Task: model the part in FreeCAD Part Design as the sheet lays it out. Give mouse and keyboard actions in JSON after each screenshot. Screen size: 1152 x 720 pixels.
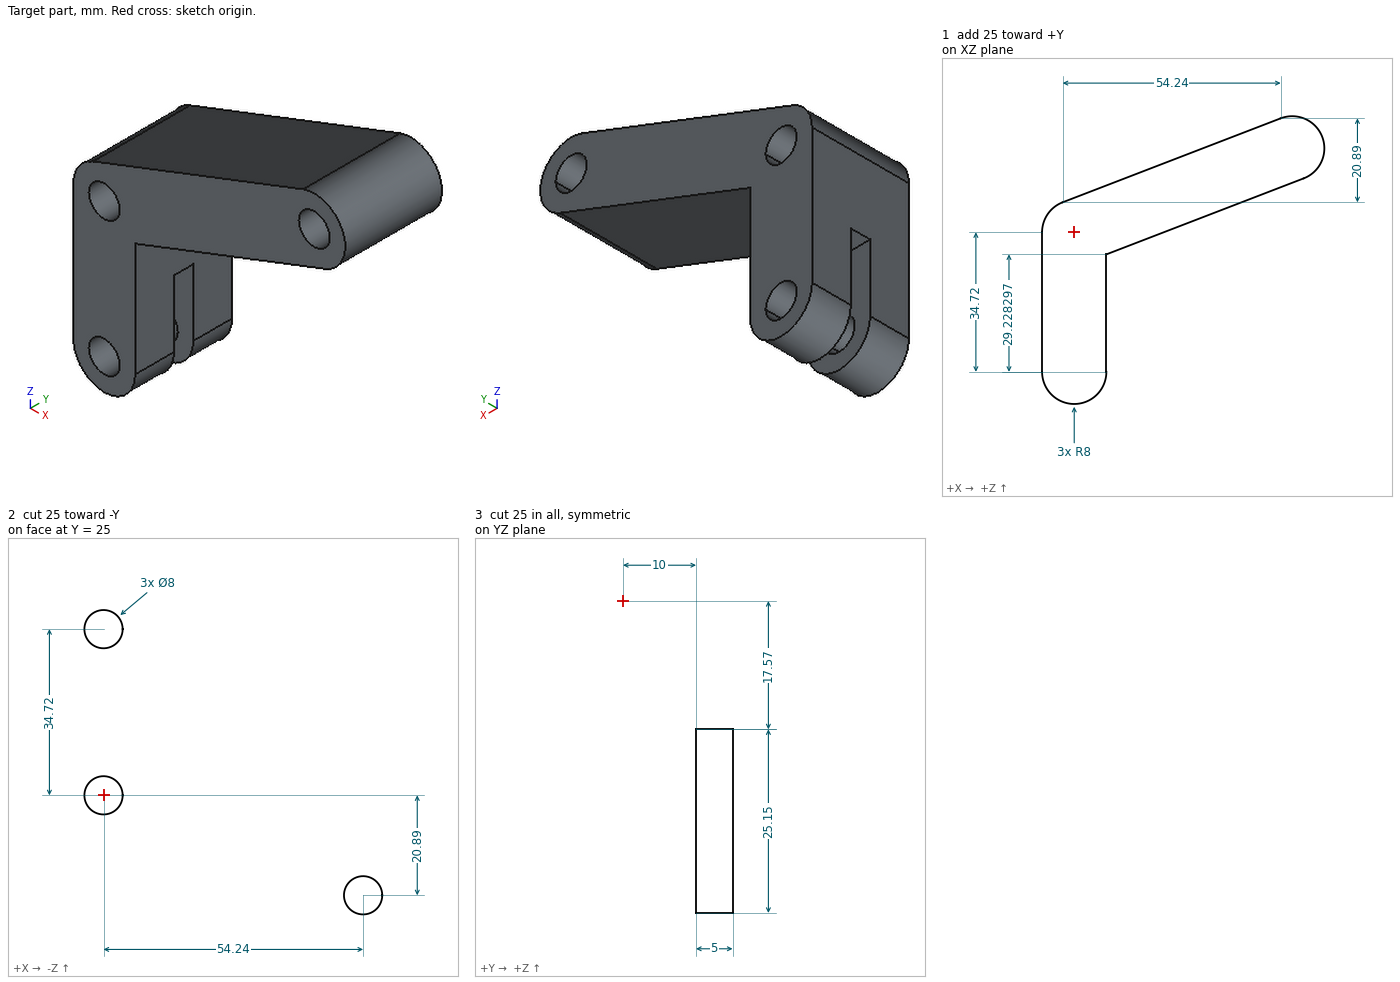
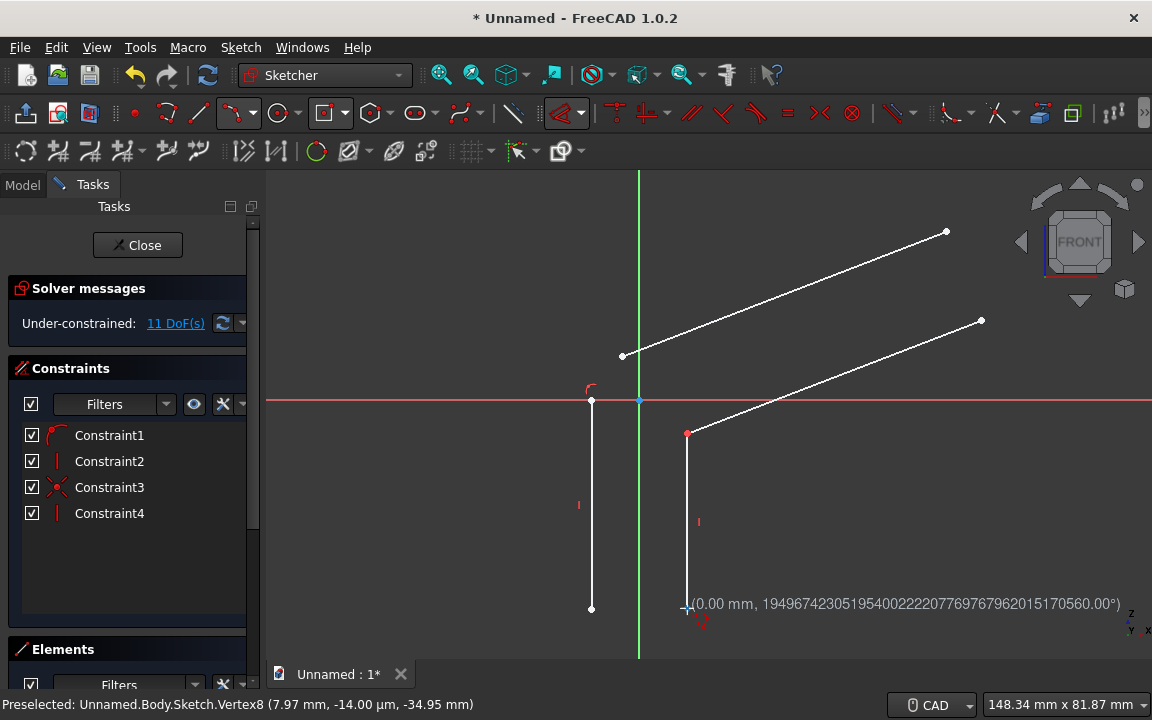
{"action": "key", "text": "g 3 a"}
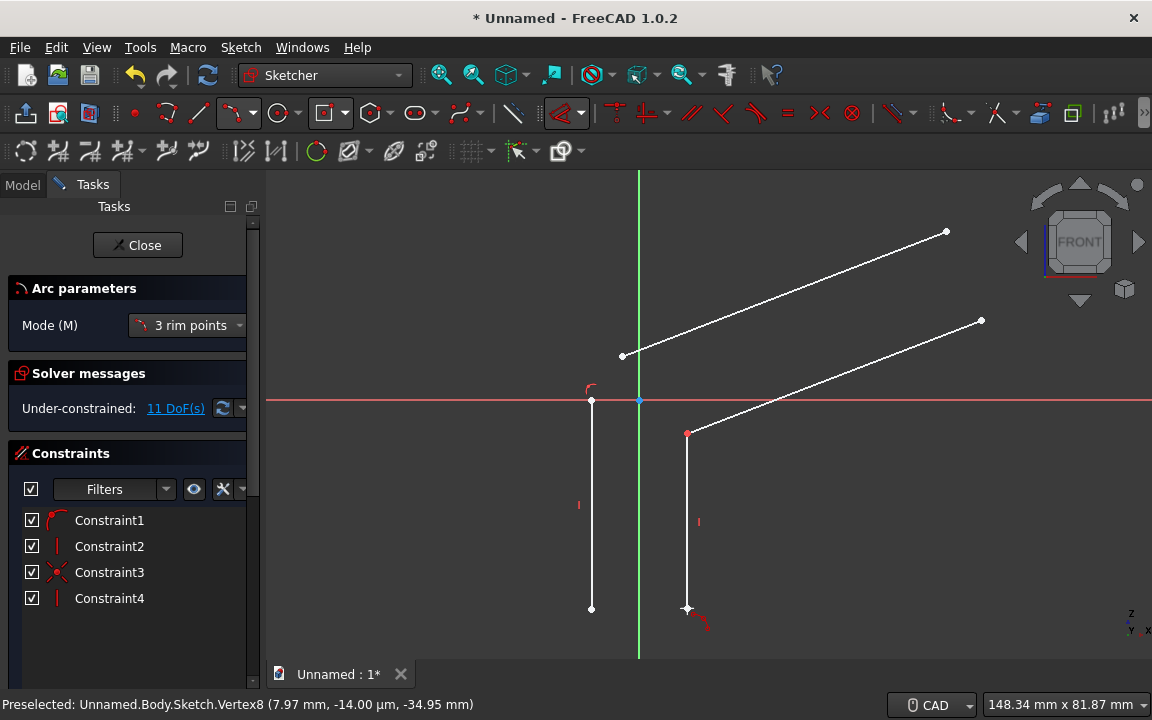
{"action": "left_click", "coordinate": [592, 400]}
{"action": "left_click", "coordinate": [622, 357]}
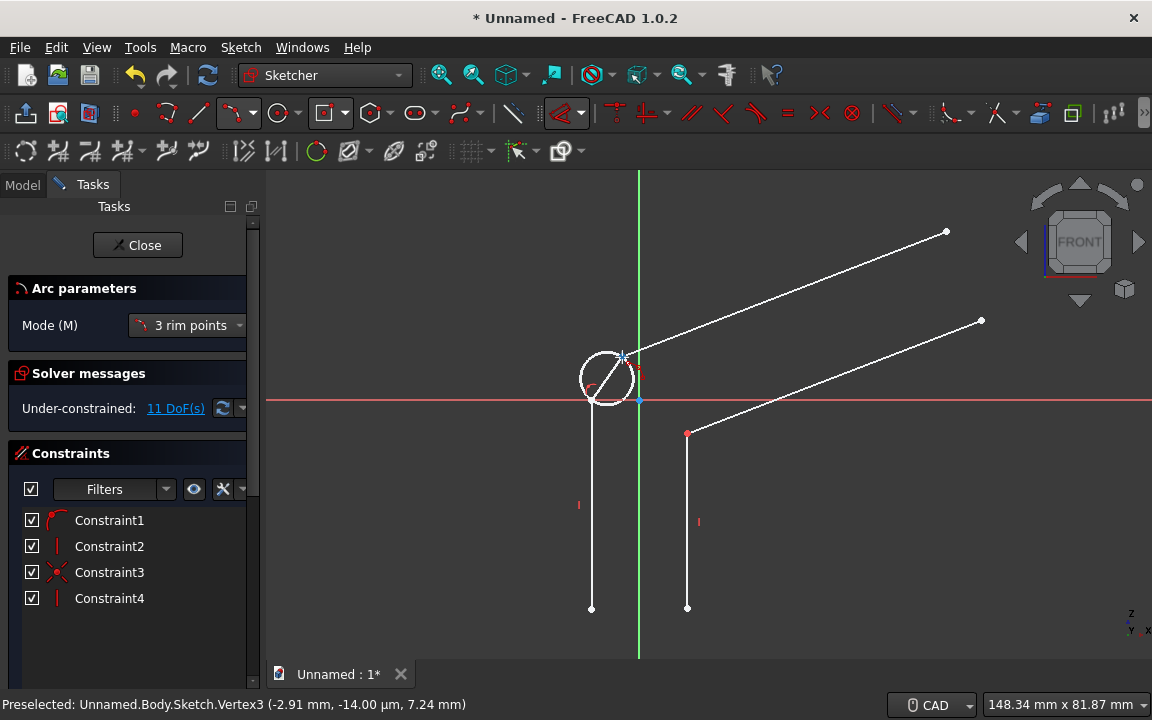
{"action": "scroll", "coordinate": [600, 373], "scroll_direction": "up", "scroll_amount": 4}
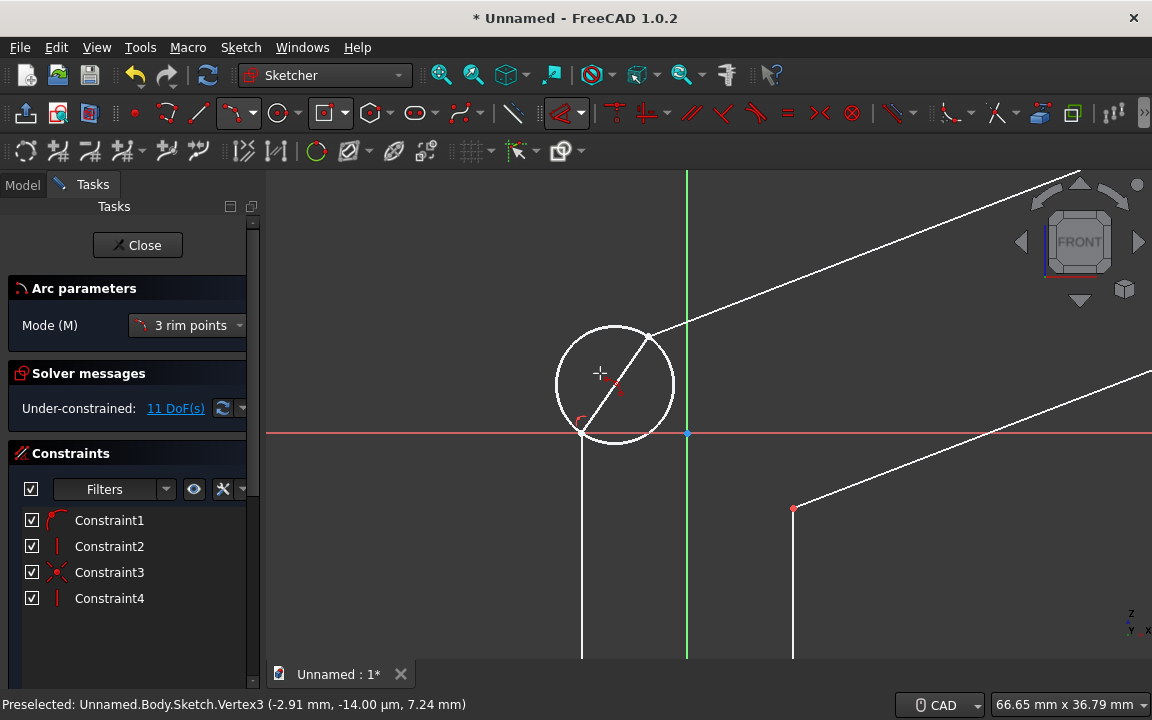
{"action": "left_click", "coordinate": [599, 373]}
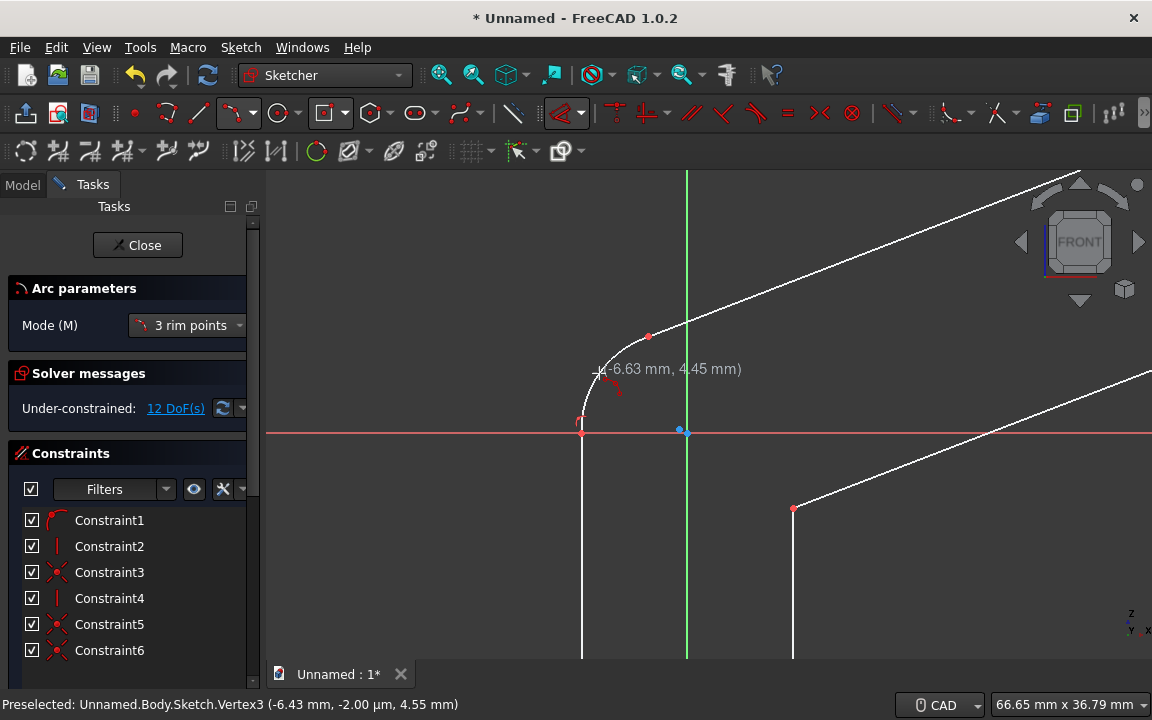
{"action": "scroll", "coordinate": [467, 365], "scroll_direction": "down", "scroll_amount": 6}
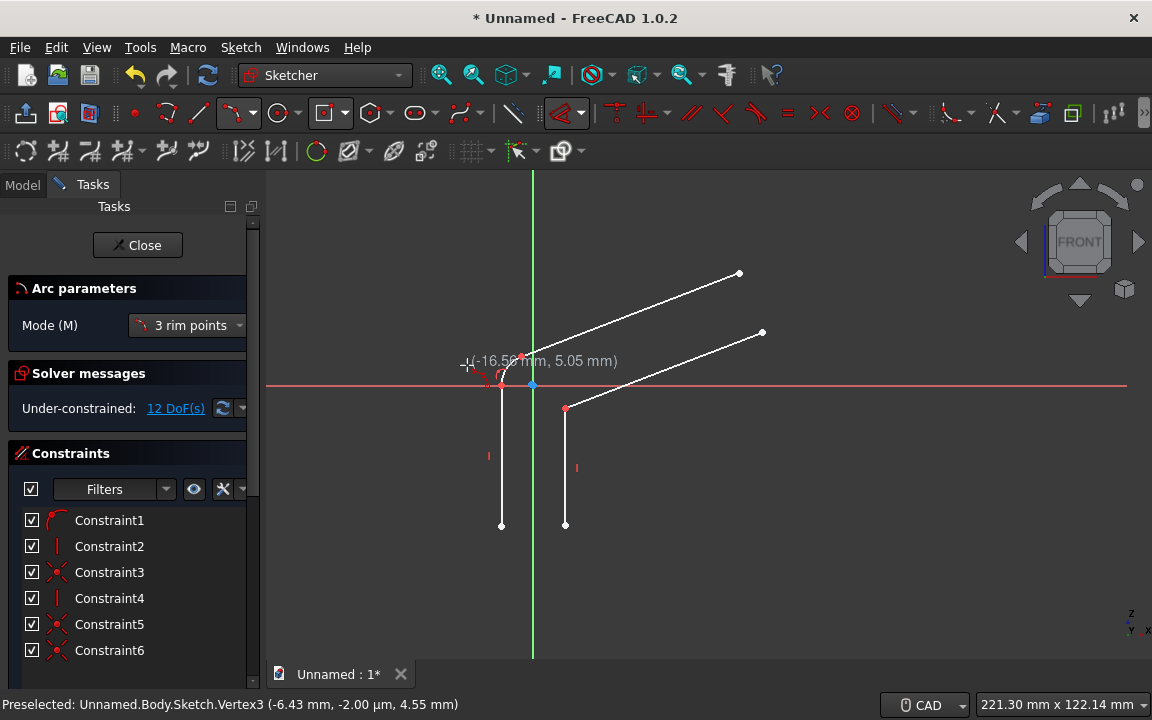
{"action": "left_click", "coordinate": [739, 273]}
{"action": "left_click", "coordinate": [762, 333]}
{"action": "left_click", "coordinate": [781, 291]}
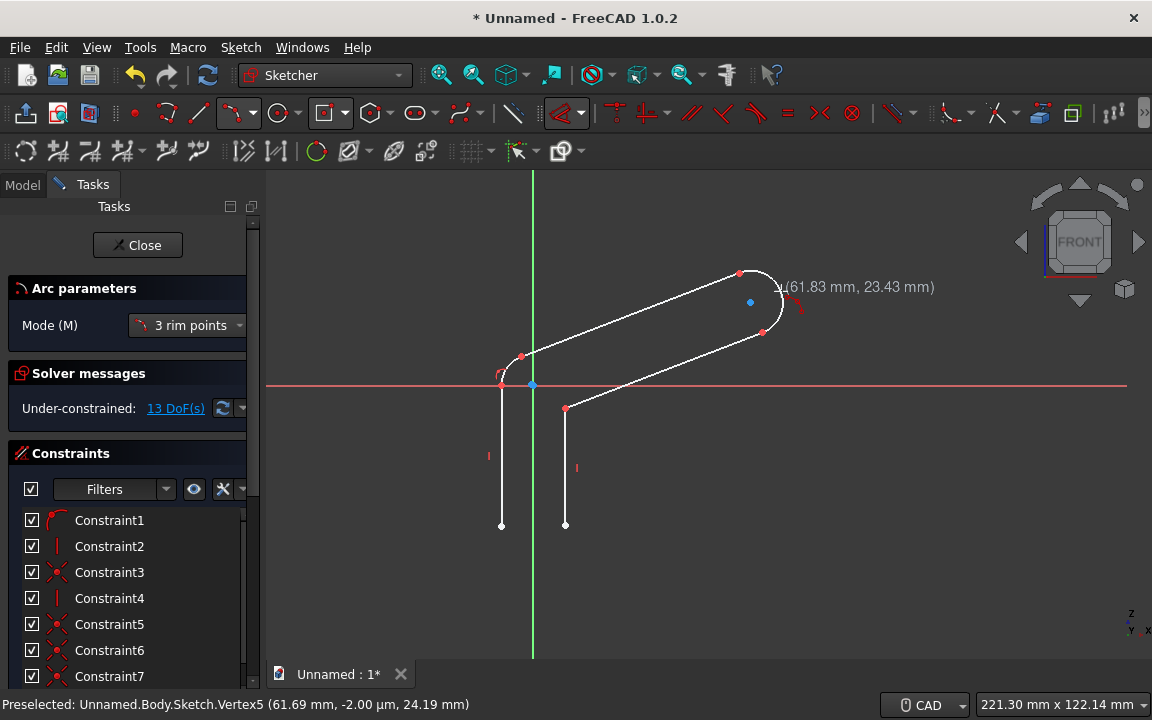
{"action": "left_click", "coordinate": [565, 526]}
{"action": "left_click", "coordinate": [502, 526]}
{"action": "left_click", "coordinate": [515, 551]}
{"action": "key", "text": "Escape"}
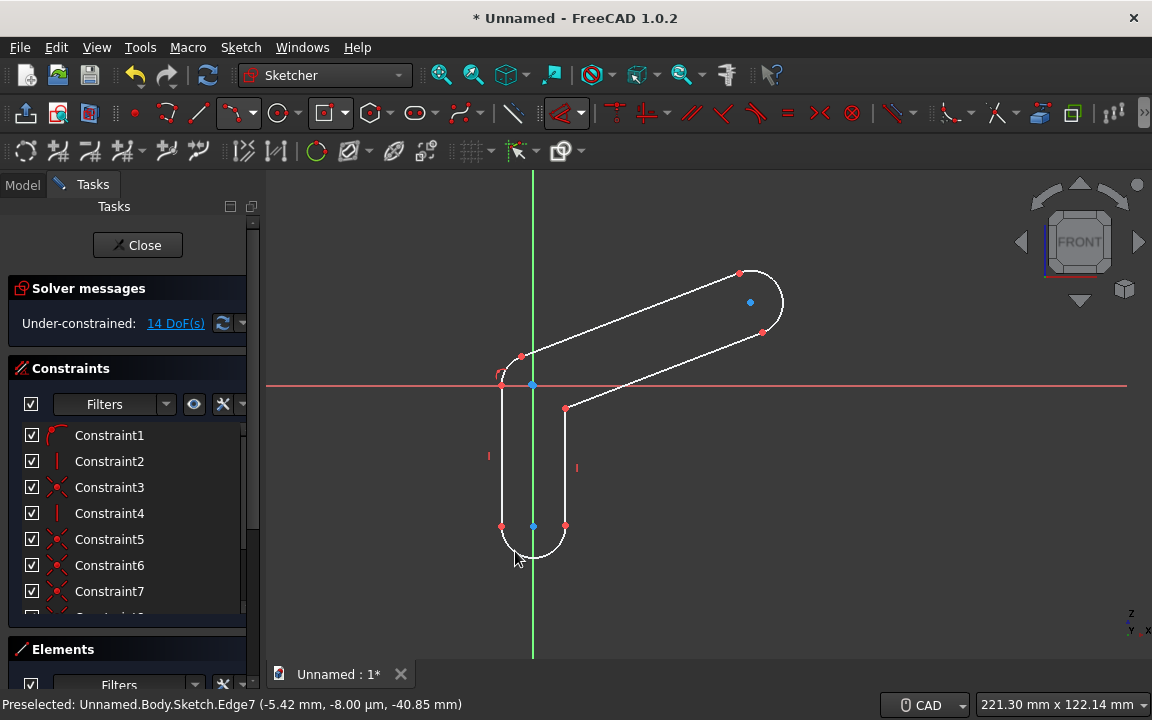
{"action": "left_click", "coordinate": [502, 484]}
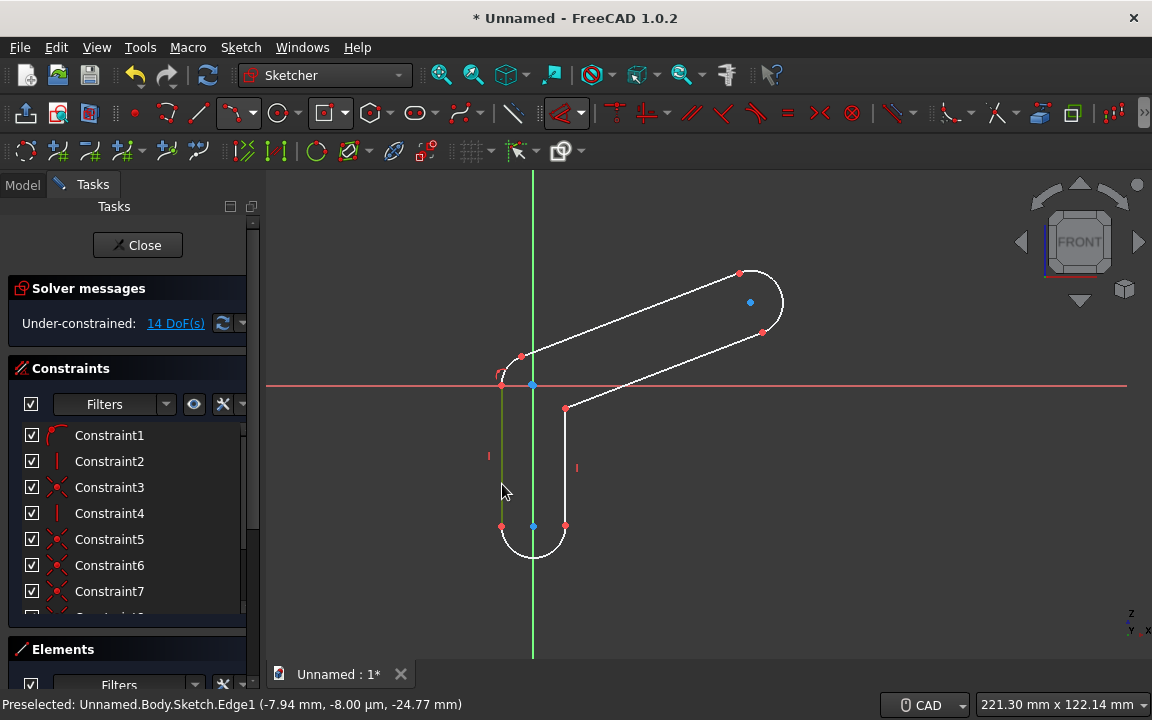
{"action": "scroll", "coordinate": [512, 362], "scroll_direction": "up", "scroll_amount": 2}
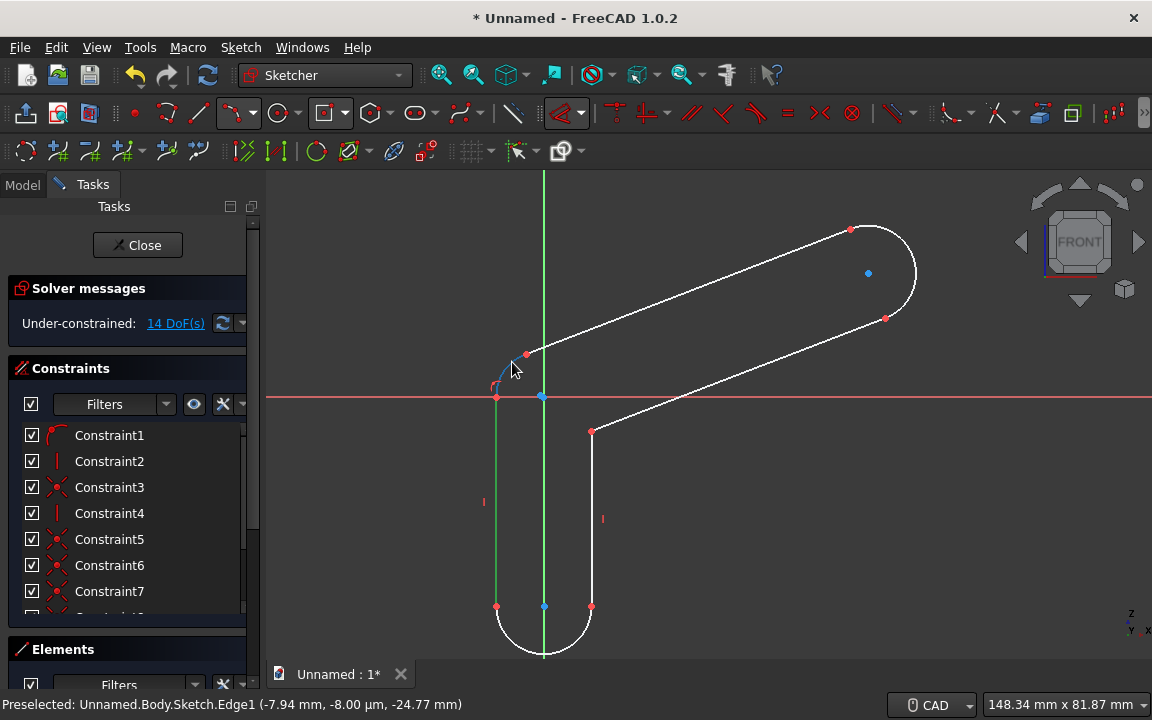
{"action": "left_click", "coordinate": [512, 362]}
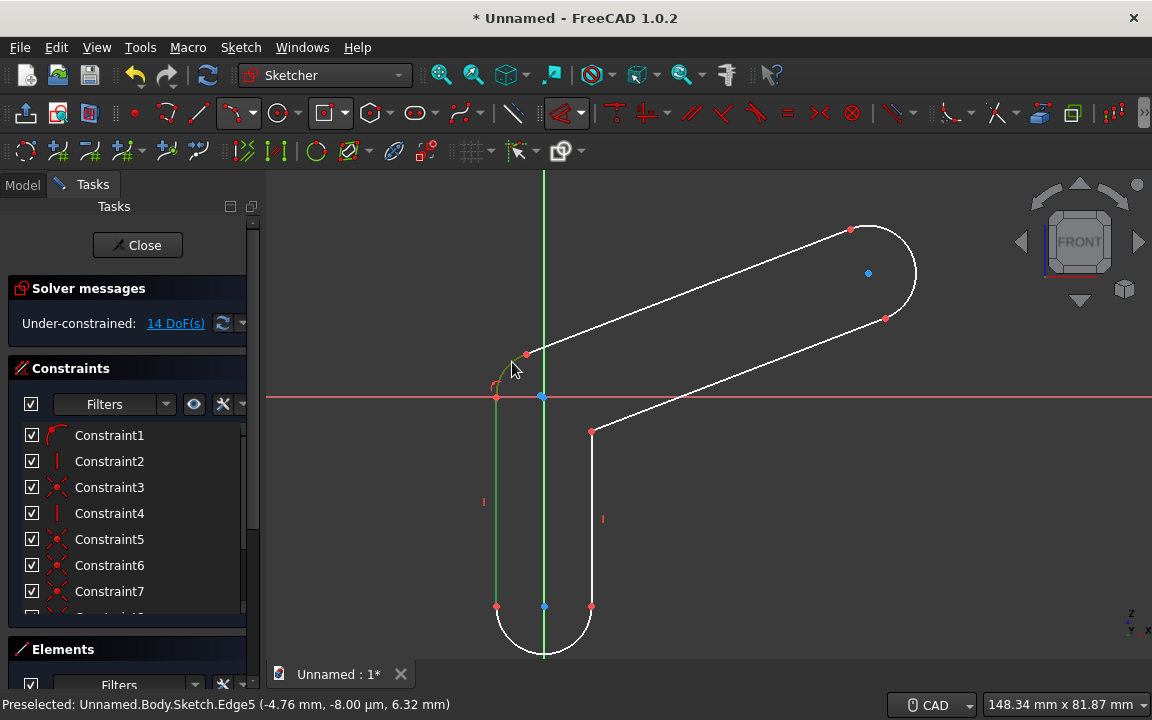
{"action": "left_click", "coordinate": [756, 114]}